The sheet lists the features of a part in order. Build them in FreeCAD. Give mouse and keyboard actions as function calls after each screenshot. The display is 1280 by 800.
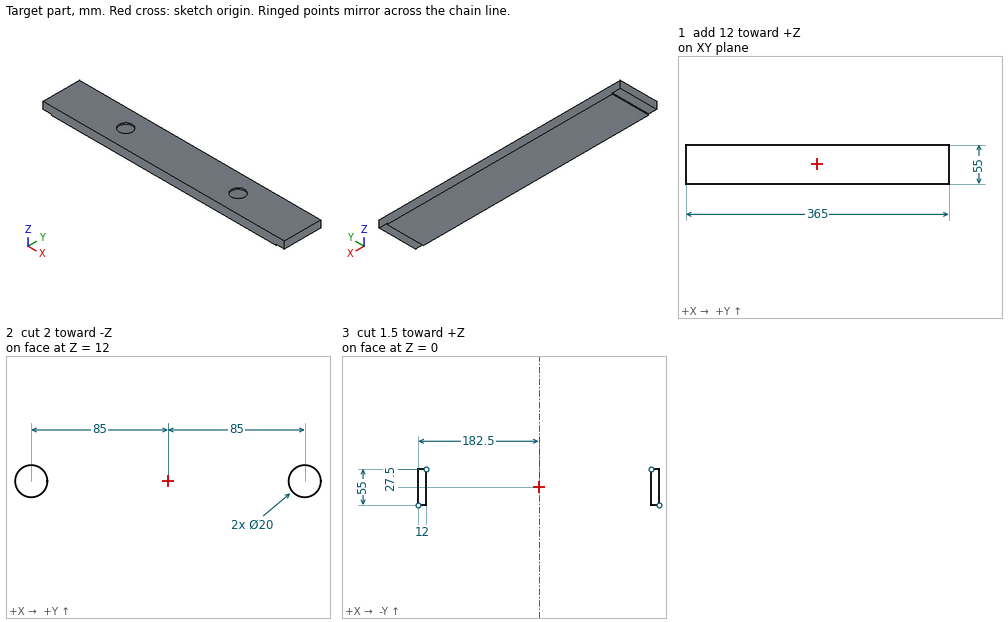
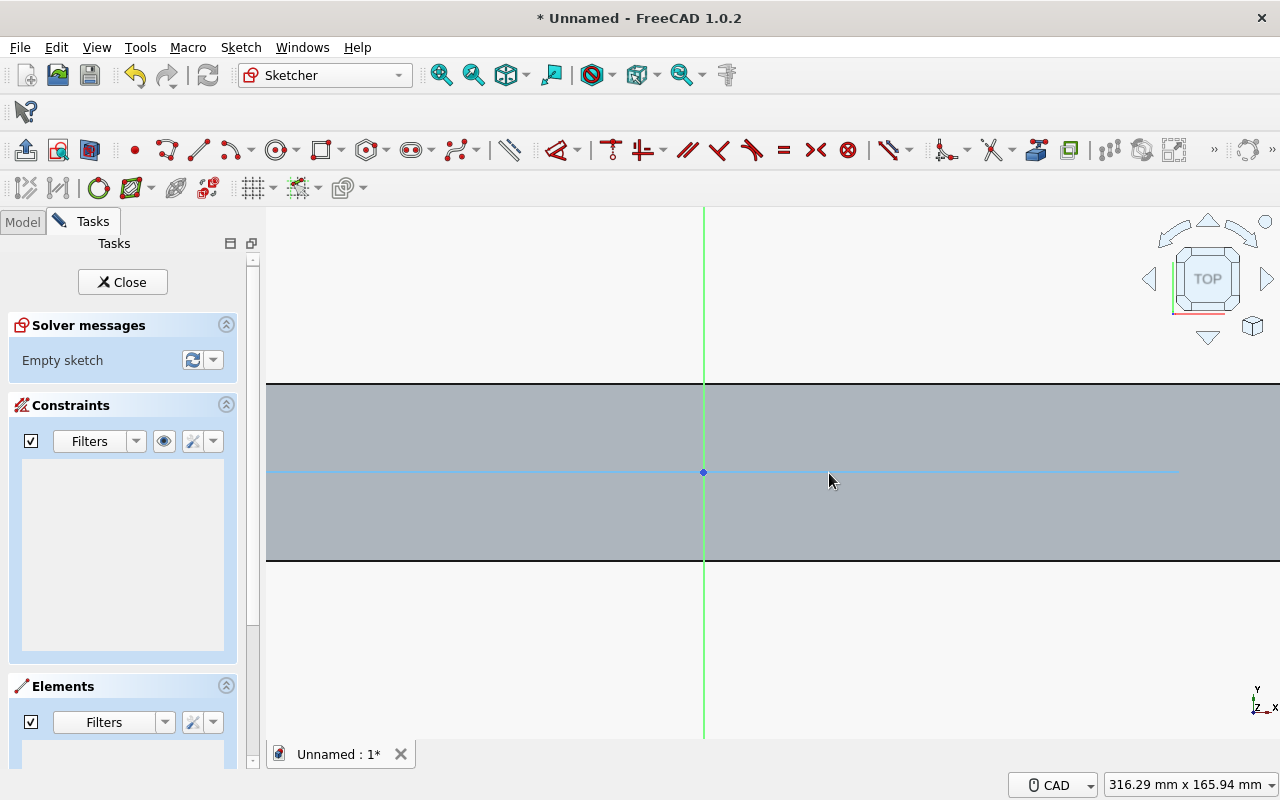
key(g)
key(c)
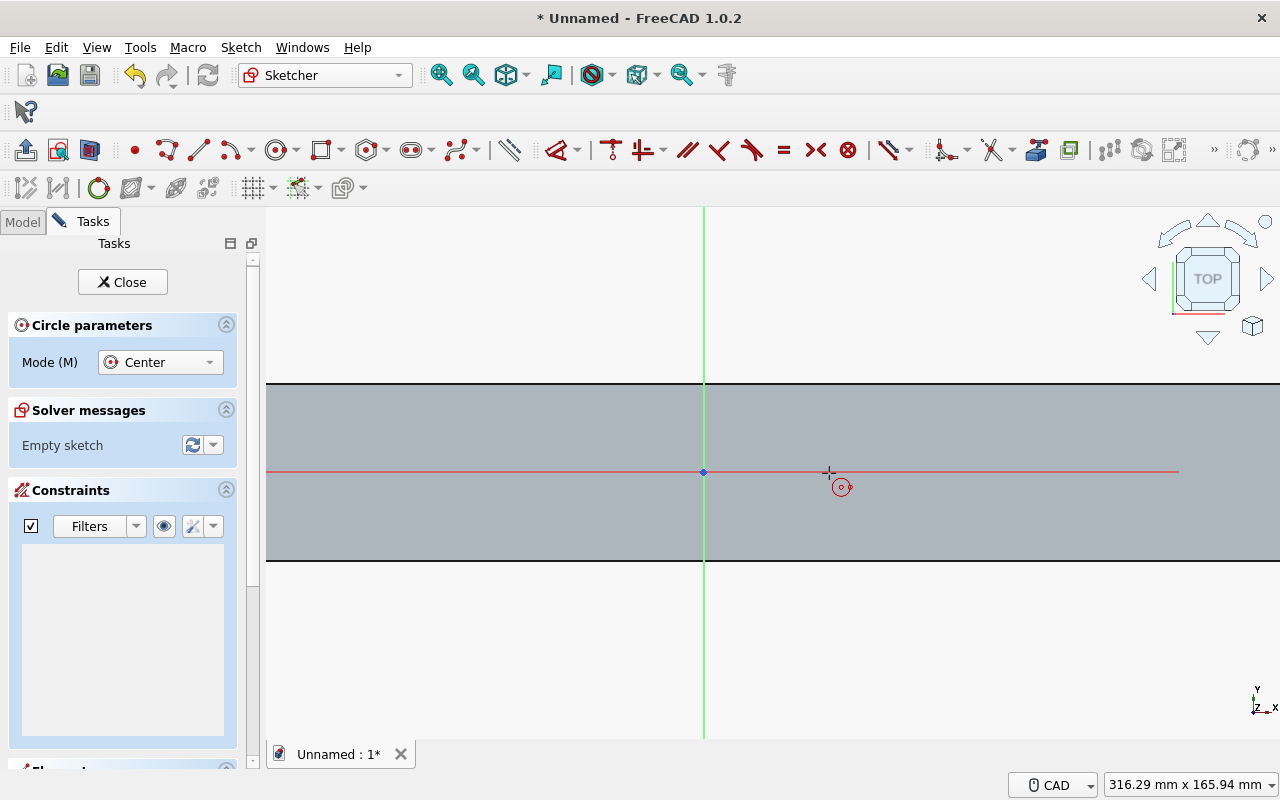
click(976, 472)
click(999, 450)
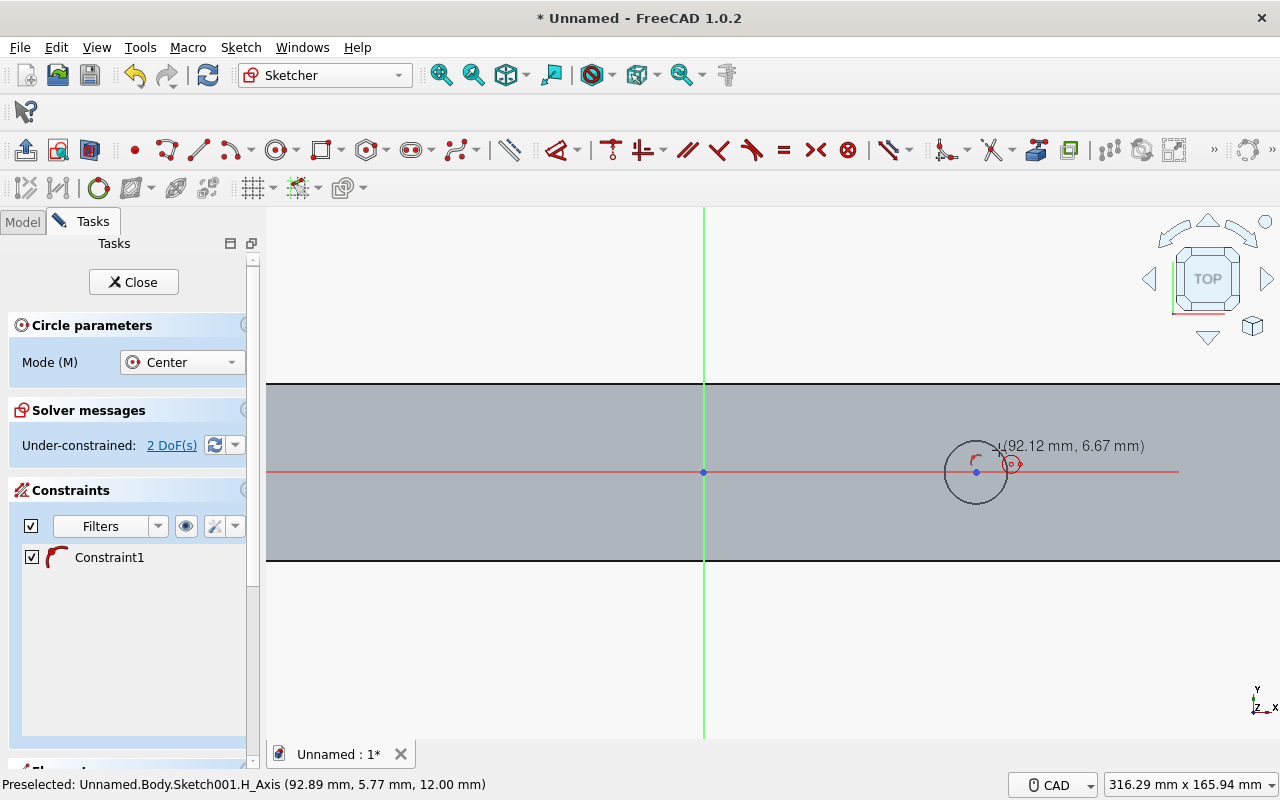
click(431, 472)
click(454, 450)
key(Escape)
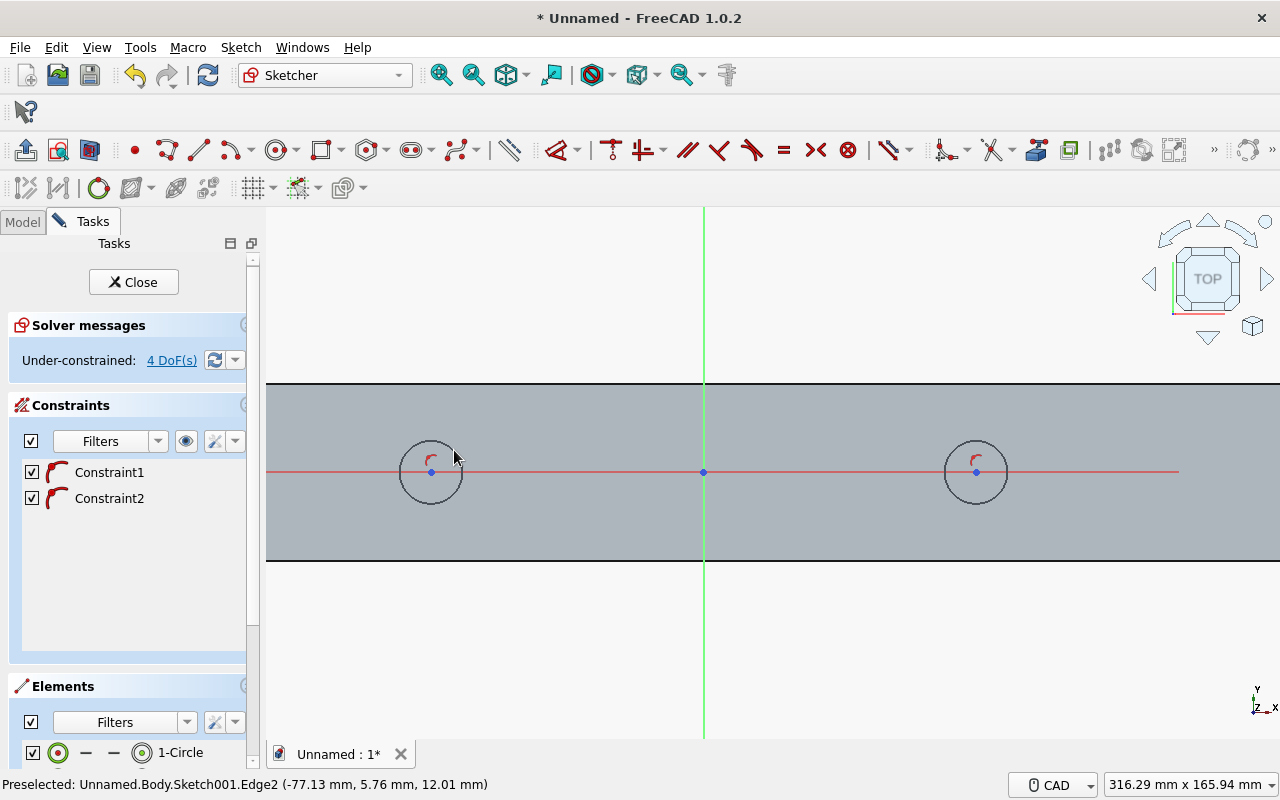
click(998, 450)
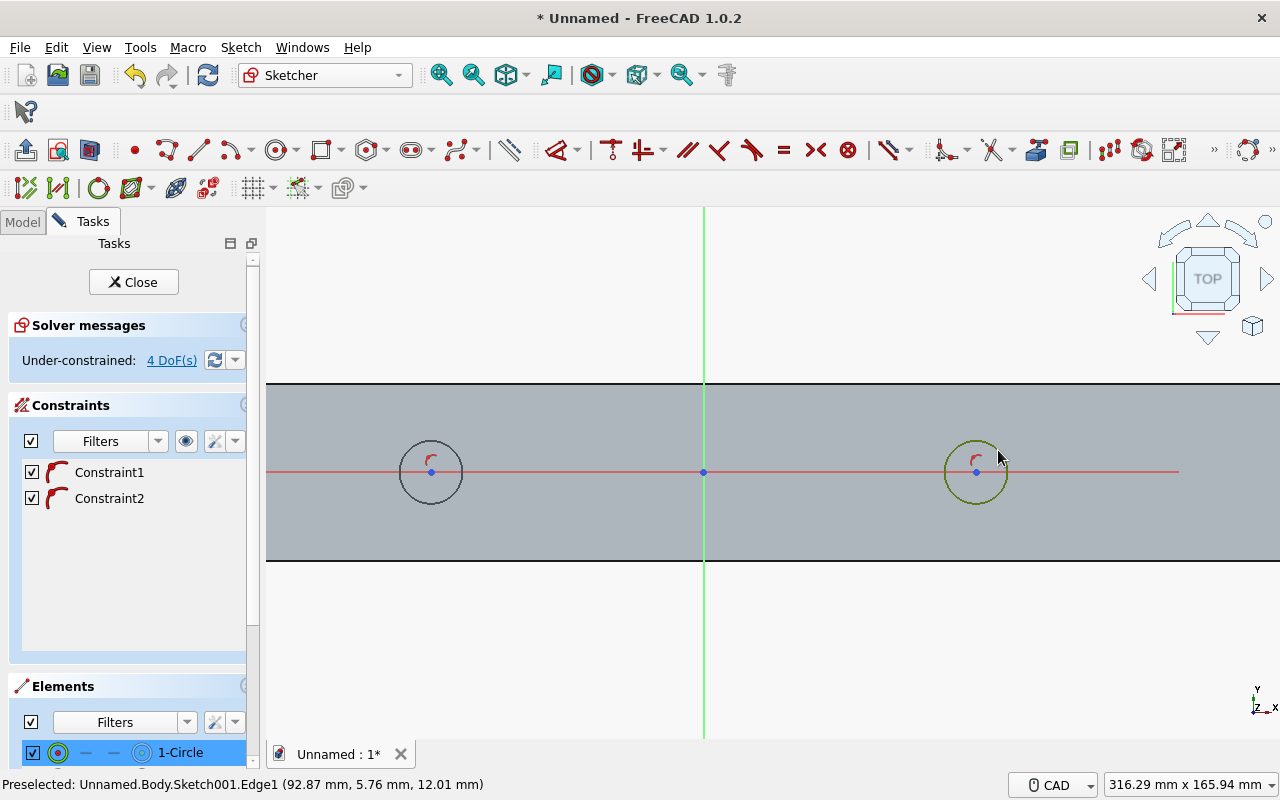
click(453, 450)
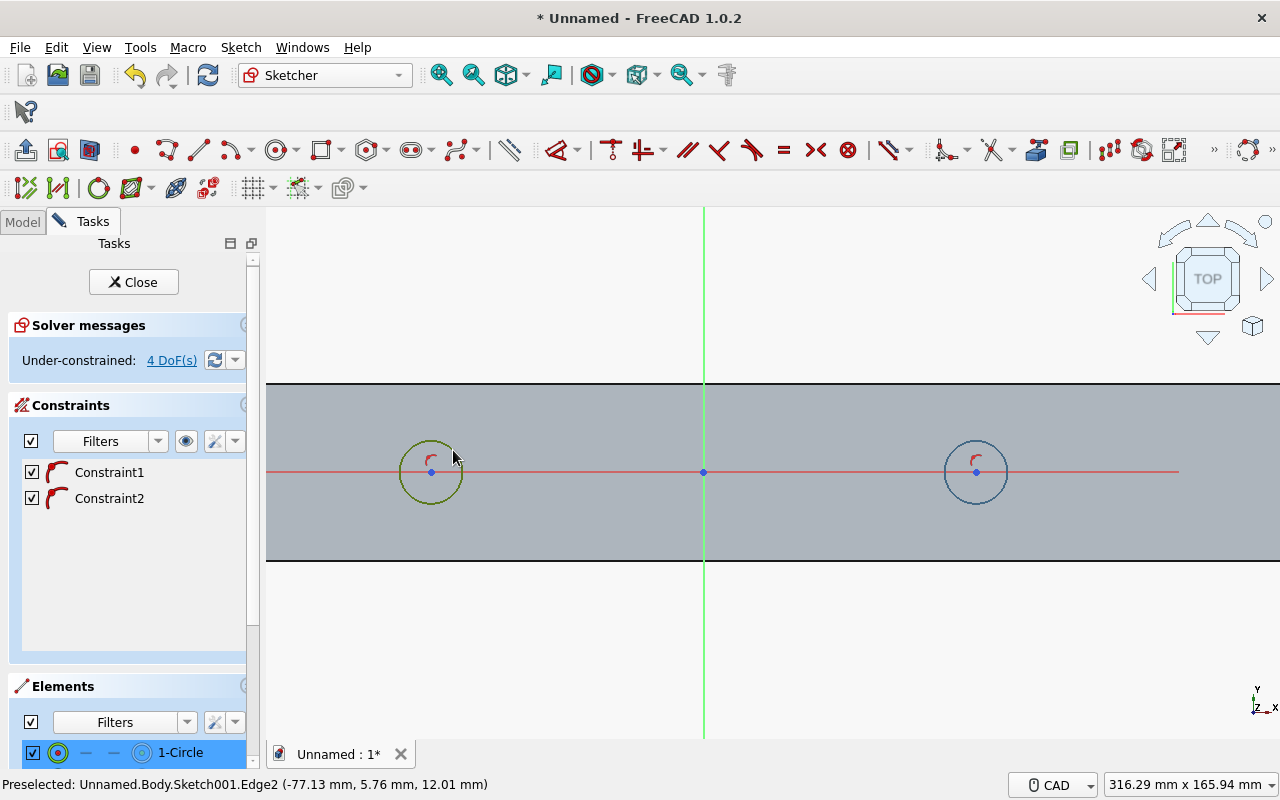
key(e)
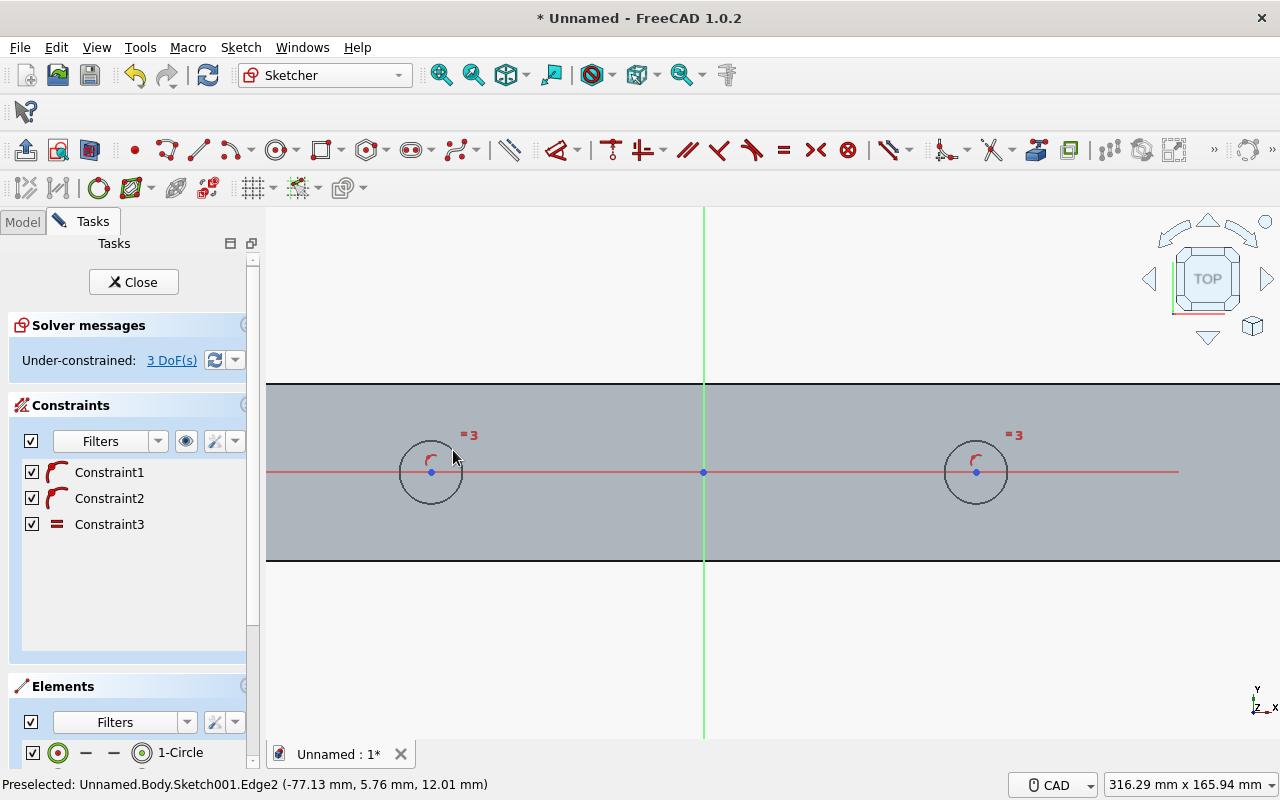
key(d)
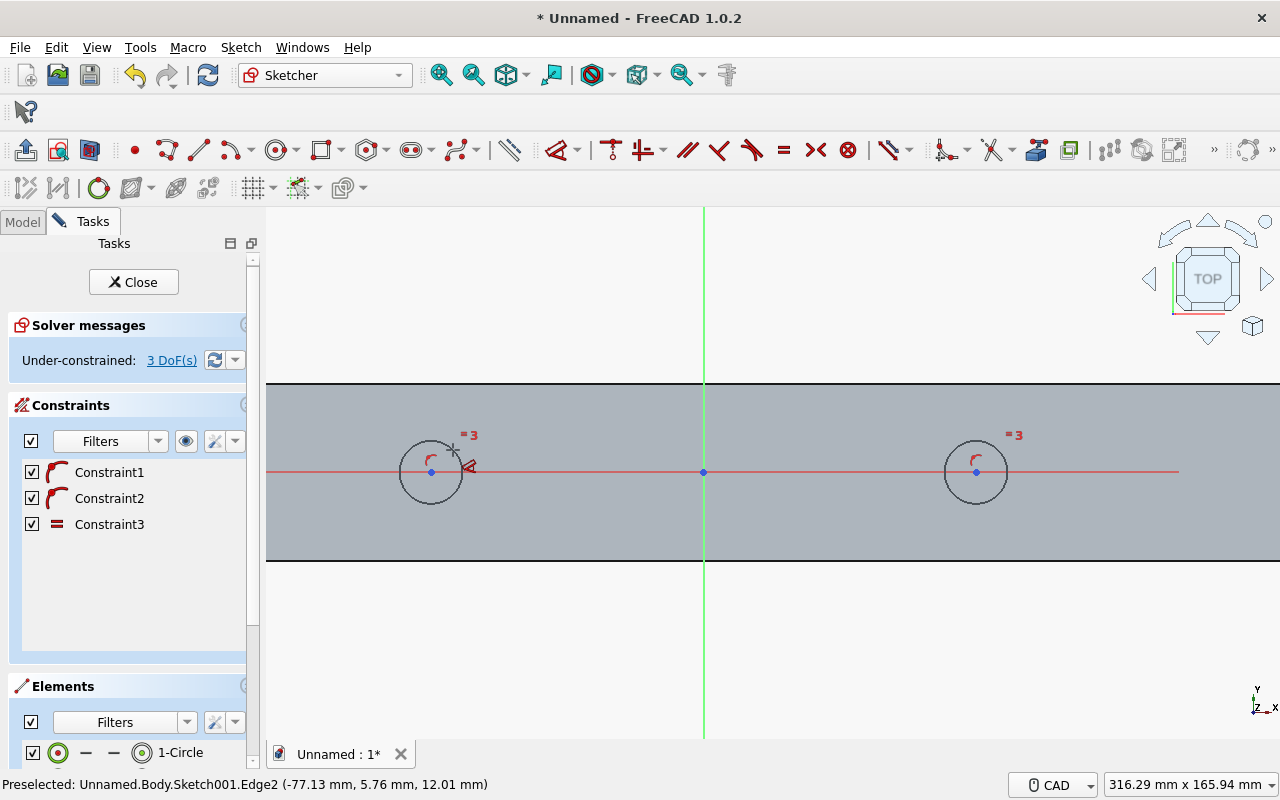
click(998, 450)
click(1020, 427)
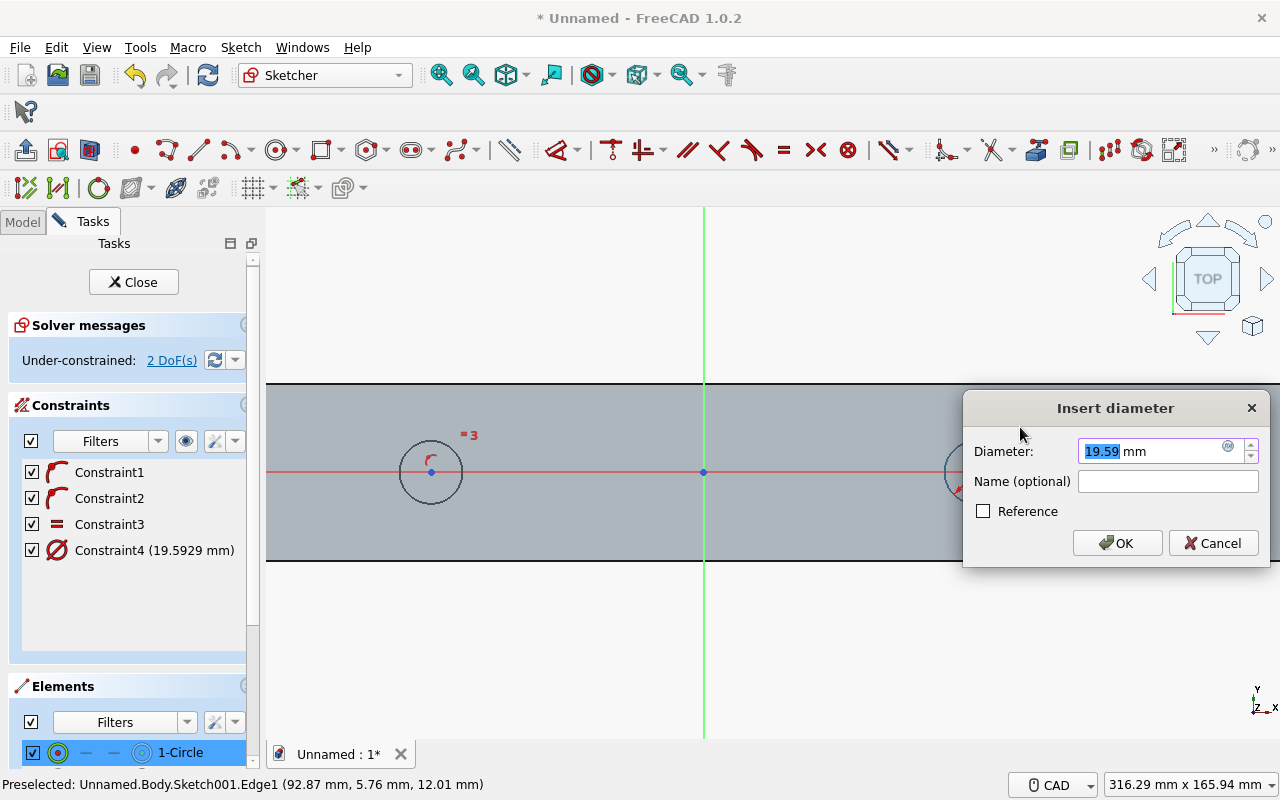
text(20)
key(Return)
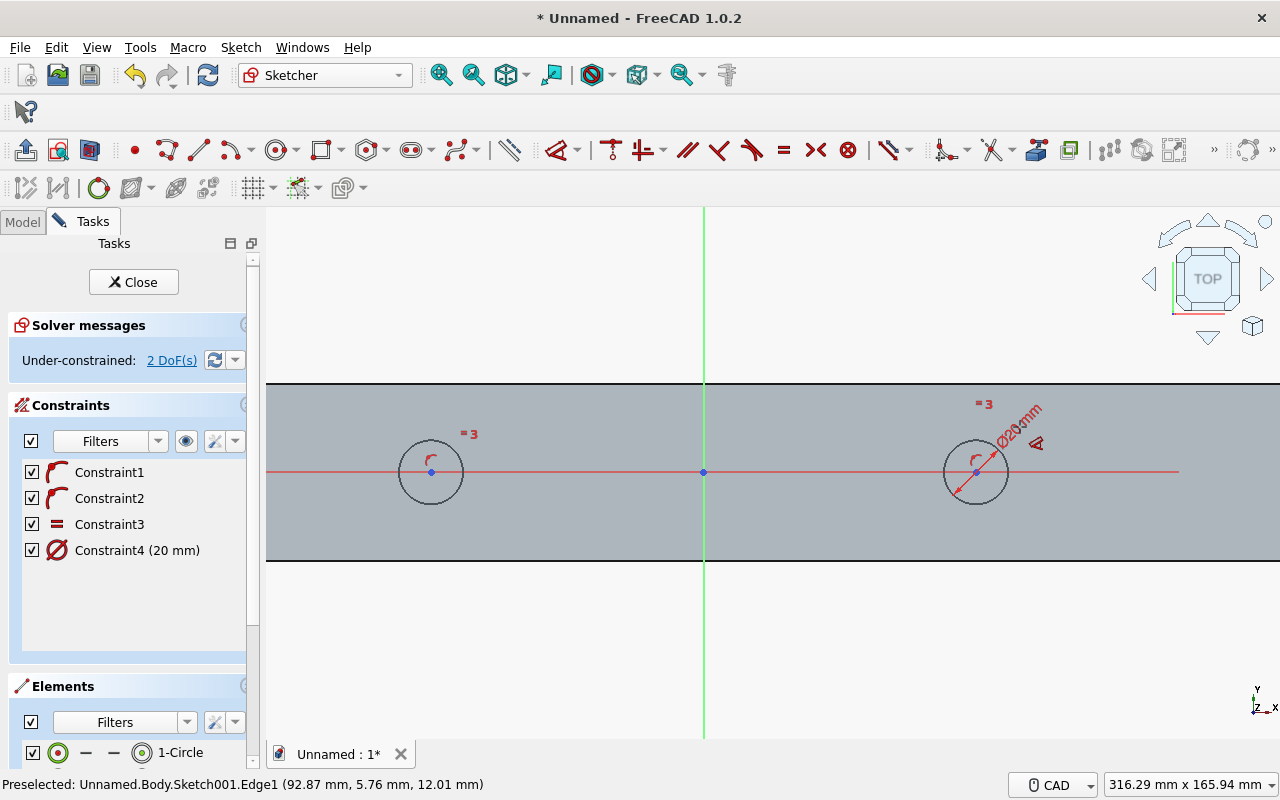
click(976, 472)
click(840, 506)